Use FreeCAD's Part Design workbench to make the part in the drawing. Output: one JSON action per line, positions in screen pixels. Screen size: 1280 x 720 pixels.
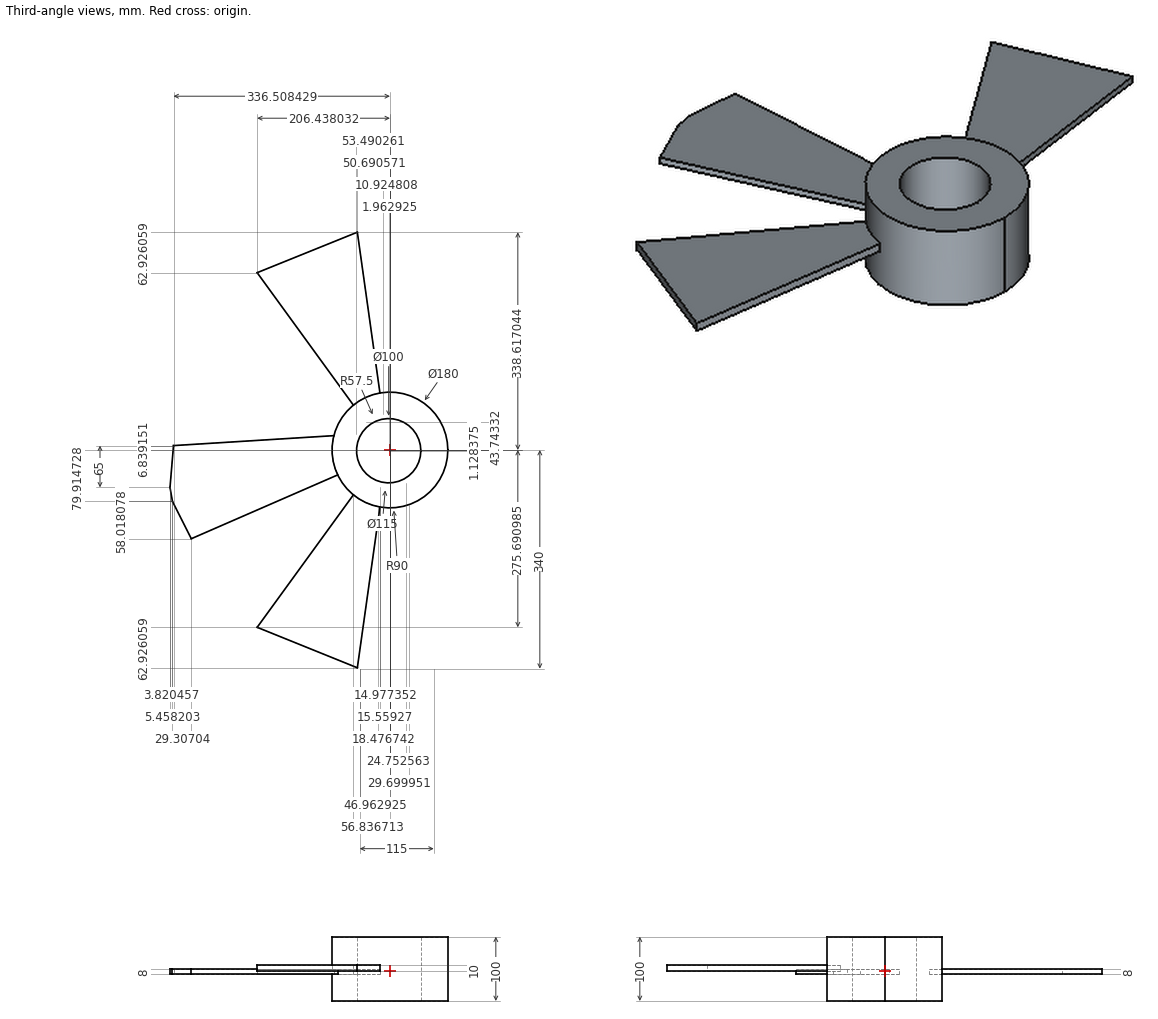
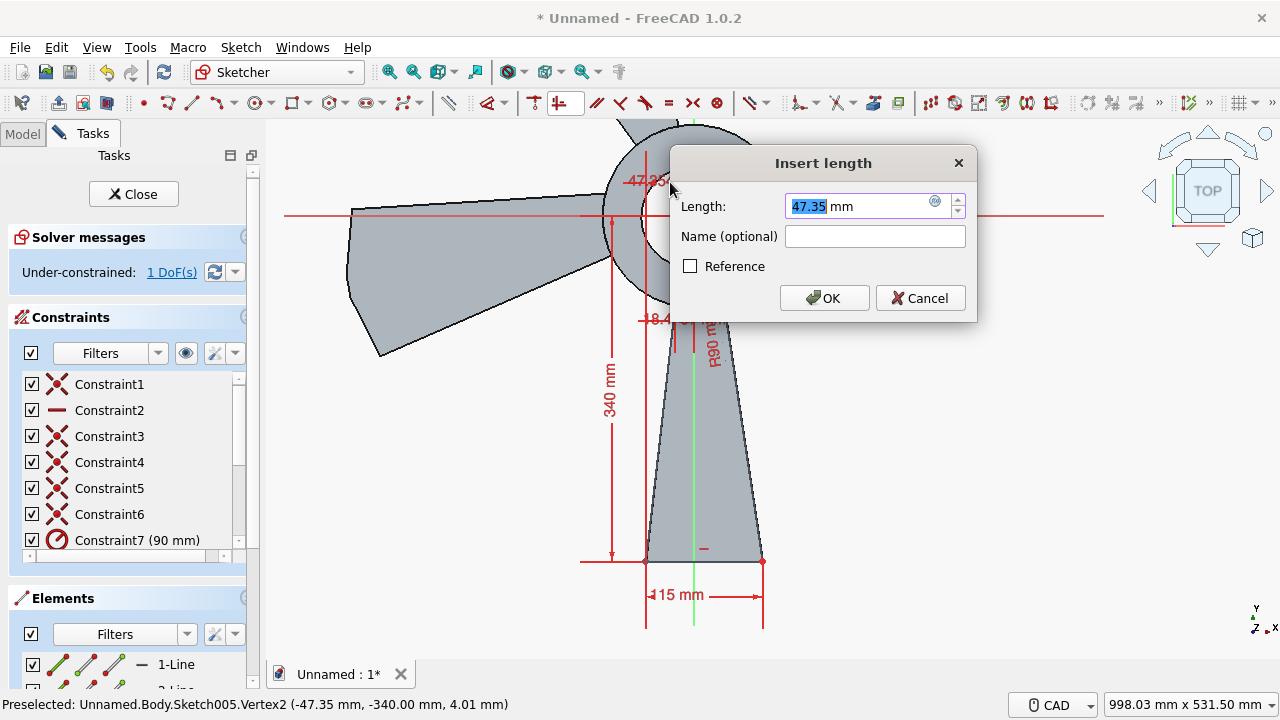
{"action": "type", "text": "46.962925"}
{"action": "key", "text": "Return"}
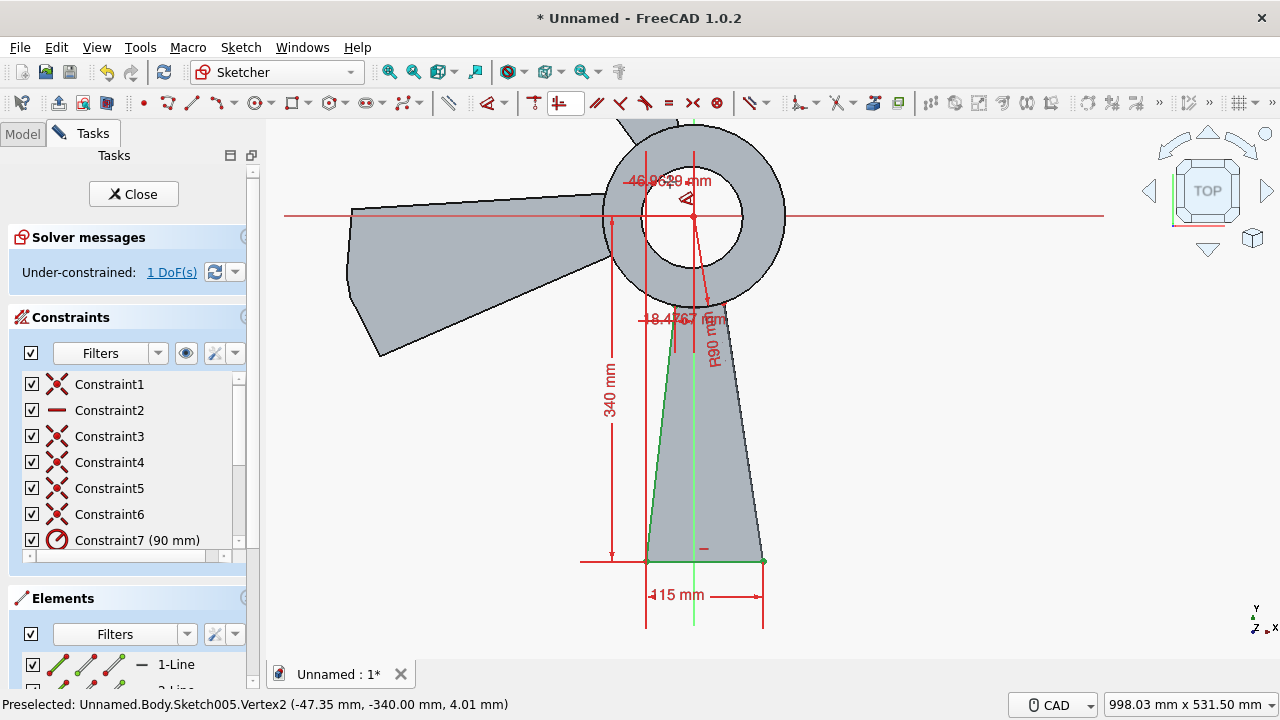
{"action": "scroll", "coordinate": [724, 303], "scroll_direction": "up", "scroll_amount": 2}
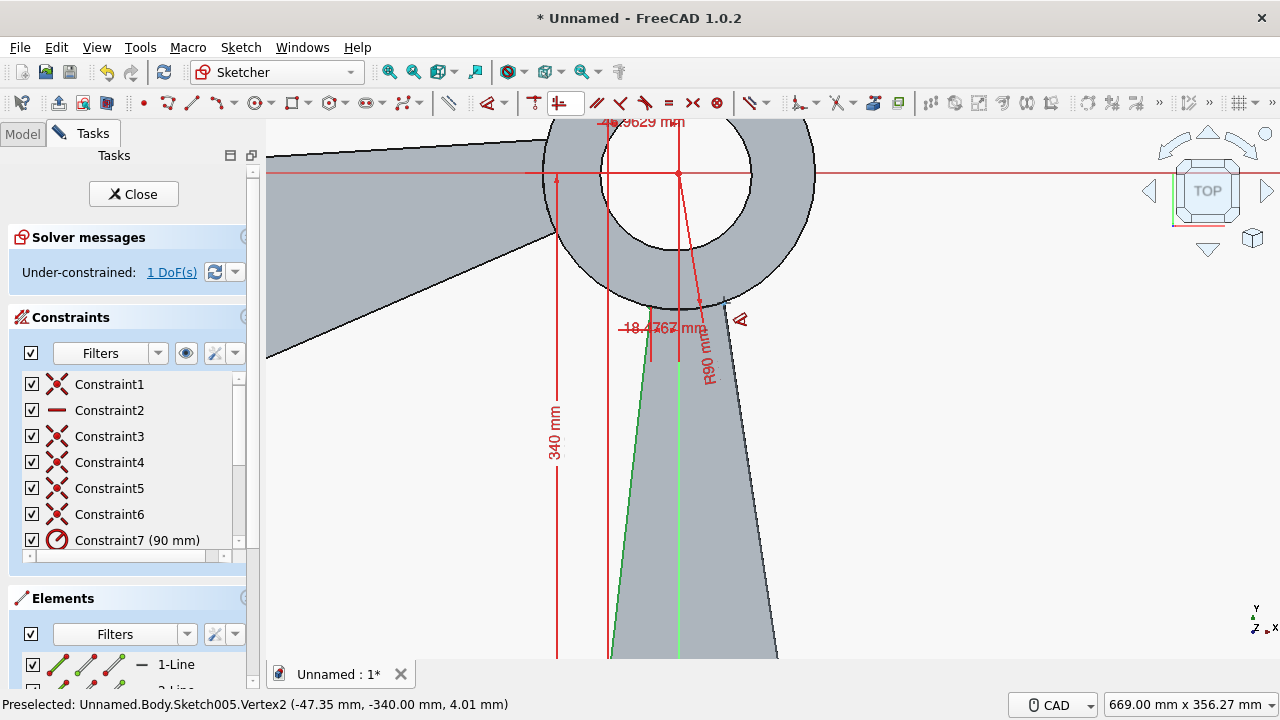
{"action": "left_click", "coordinate": [723, 302]}
{"action": "left_click", "coordinate": [701, 384]}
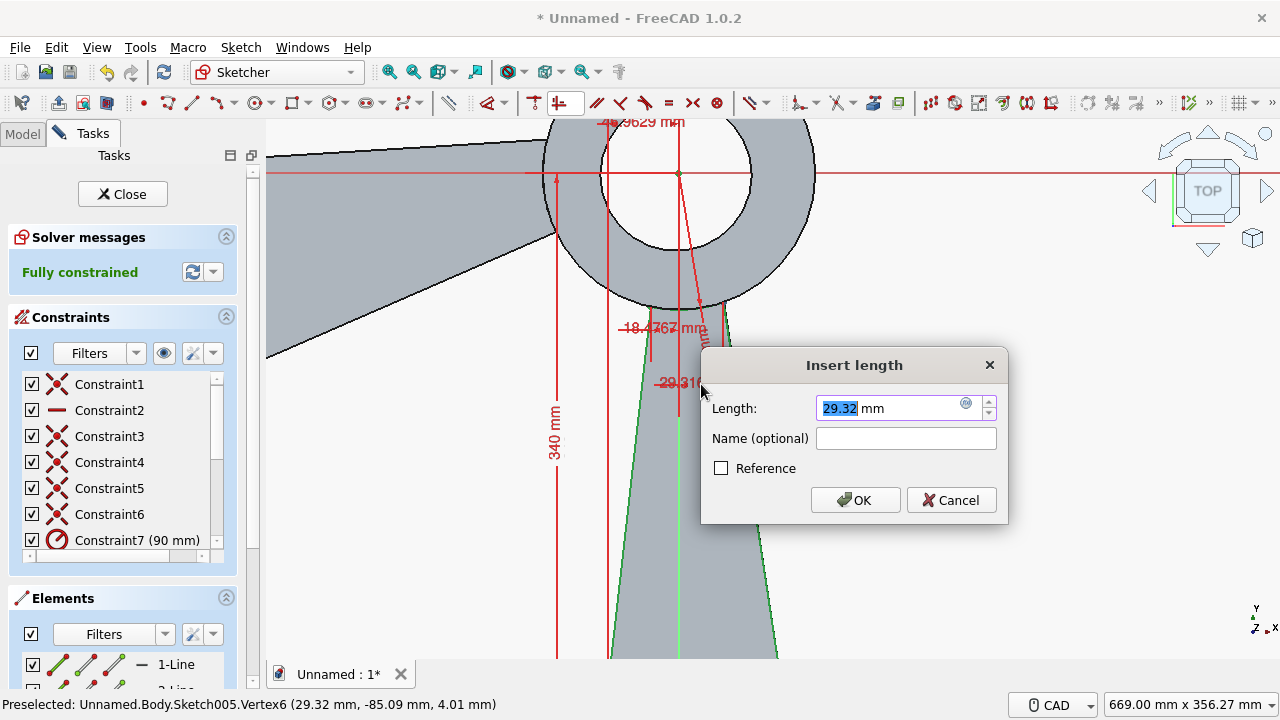
{"action": "type", "text": "29.699951"}
{"action": "key", "text": "Return"}
{"action": "key", "text": "Escape"}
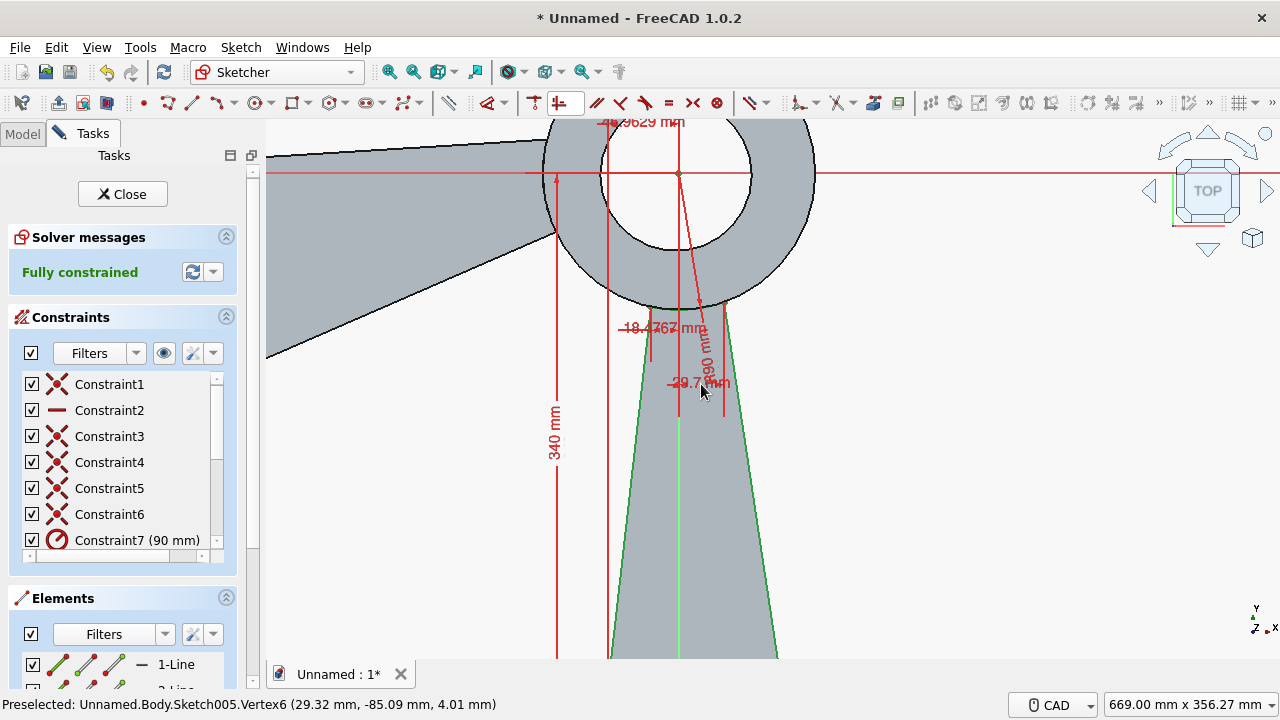
{"action": "left_click", "coordinate": [123, 194]}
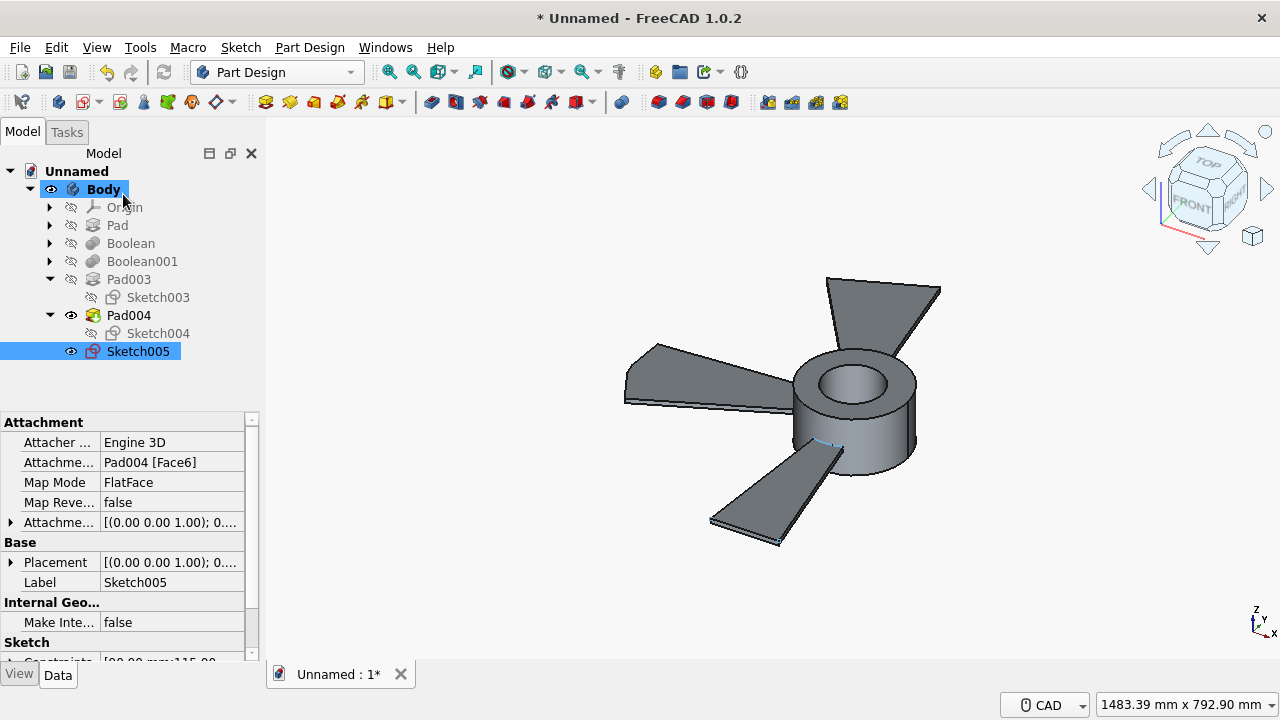
{"action": "left_click", "coordinate": [432, 102]}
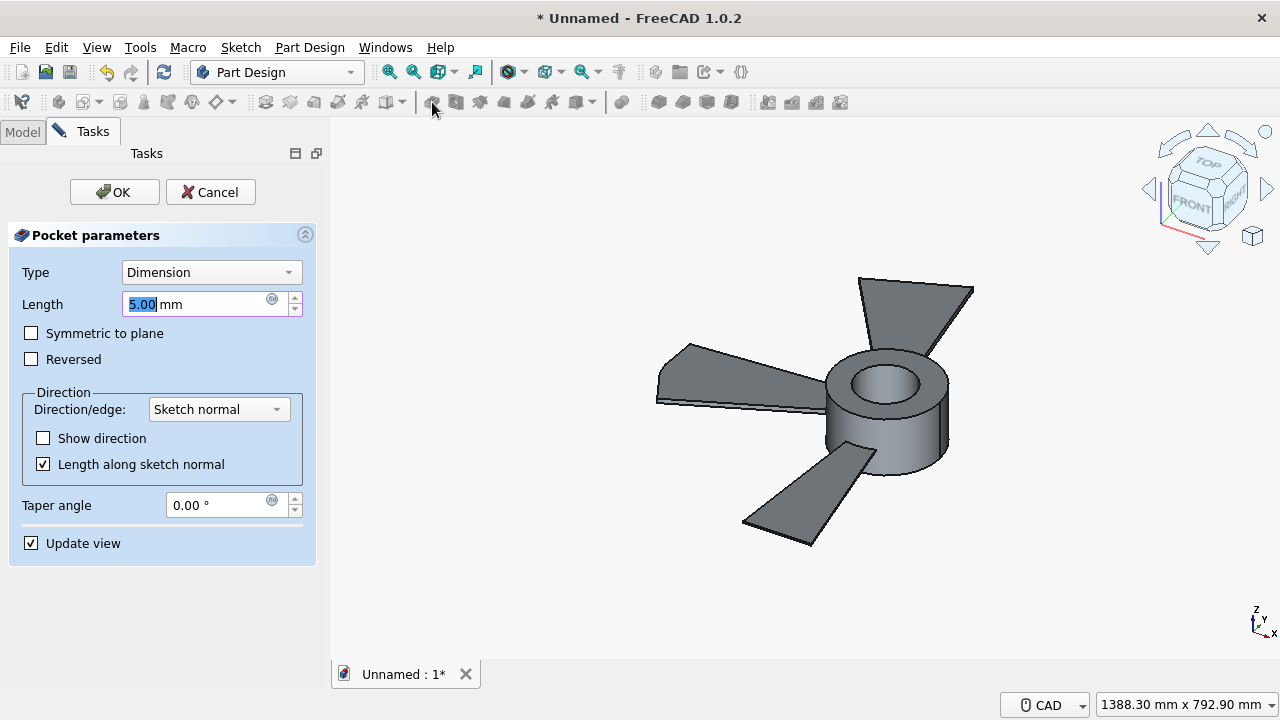
{"action": "left_click", "coordinate": [212, 272]}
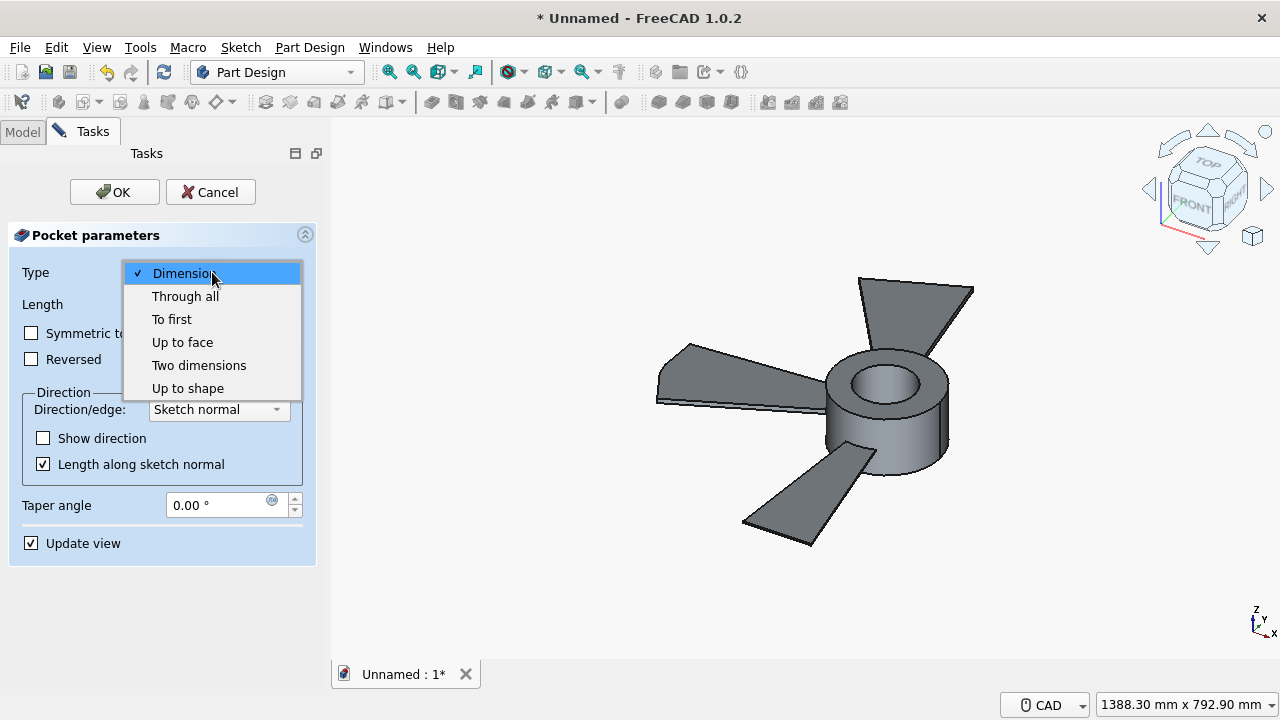
{"action": "left_click", "coordinate": [212, 296]}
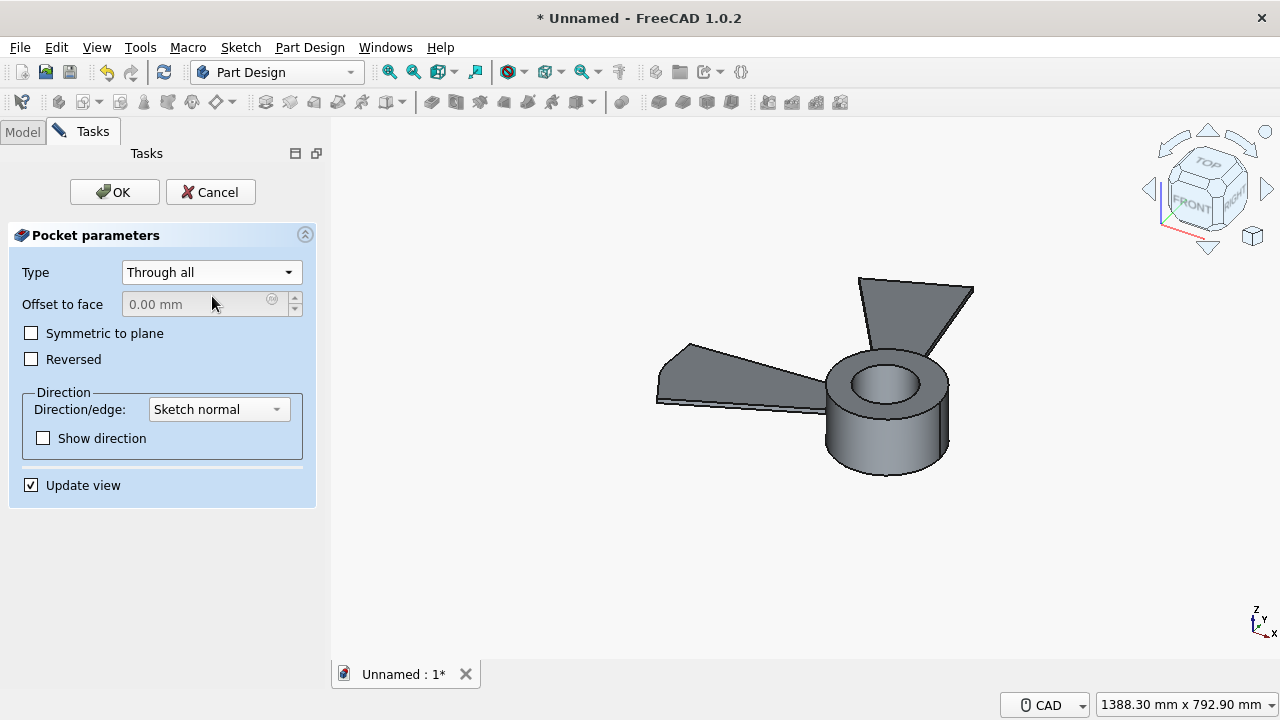
{"action": "left_click", "coordinate": [115, 192]}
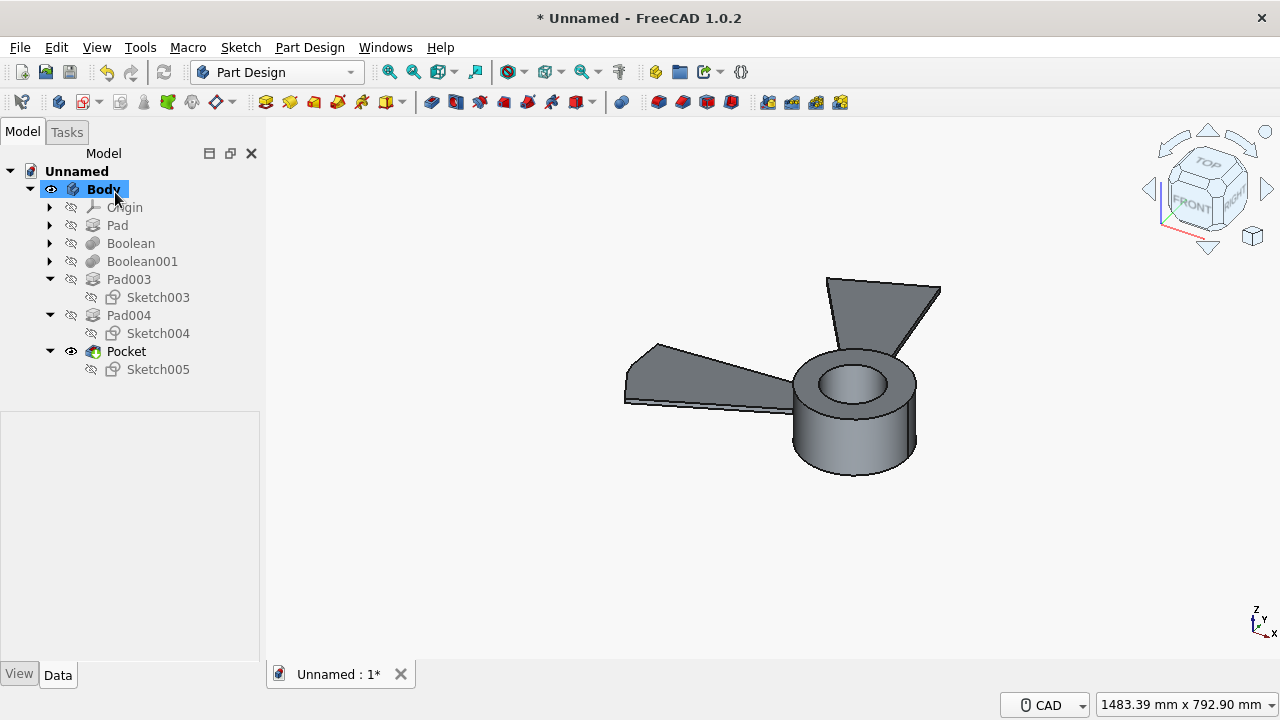
{"action": "left_click", "coordinate": [50, 207]}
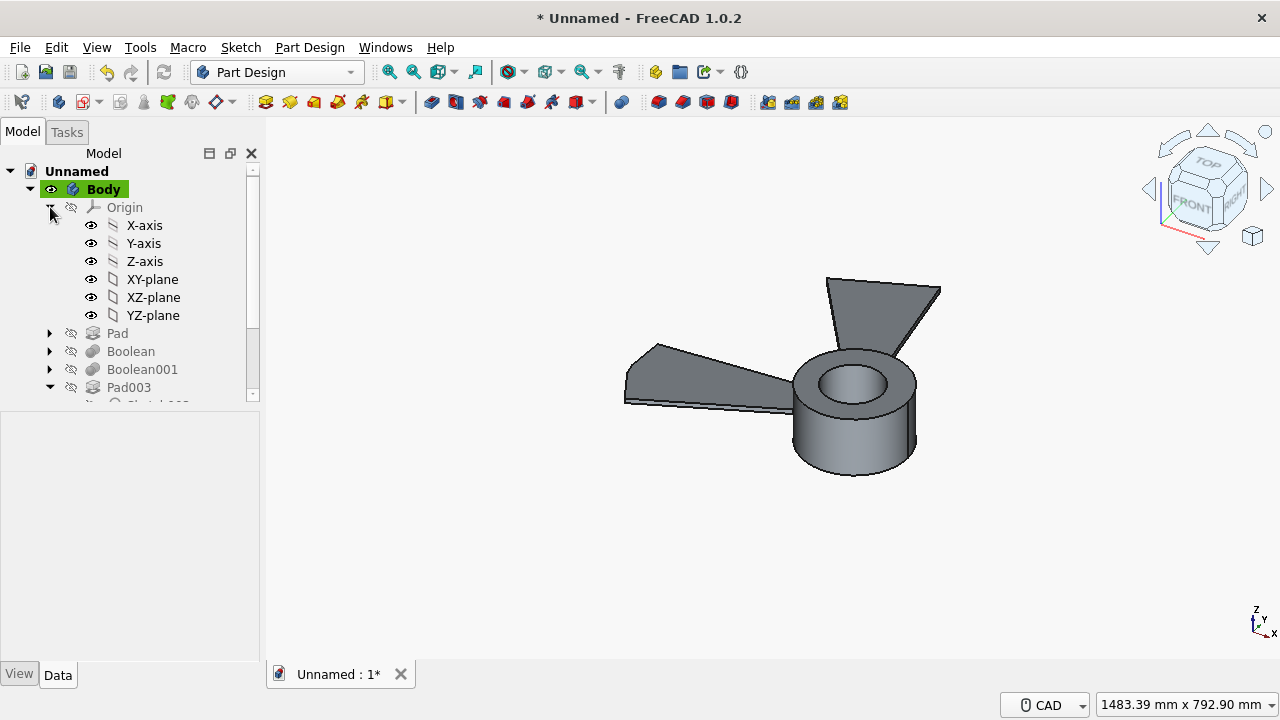
{"action": "left_click", "coordinate": [136, 279]}